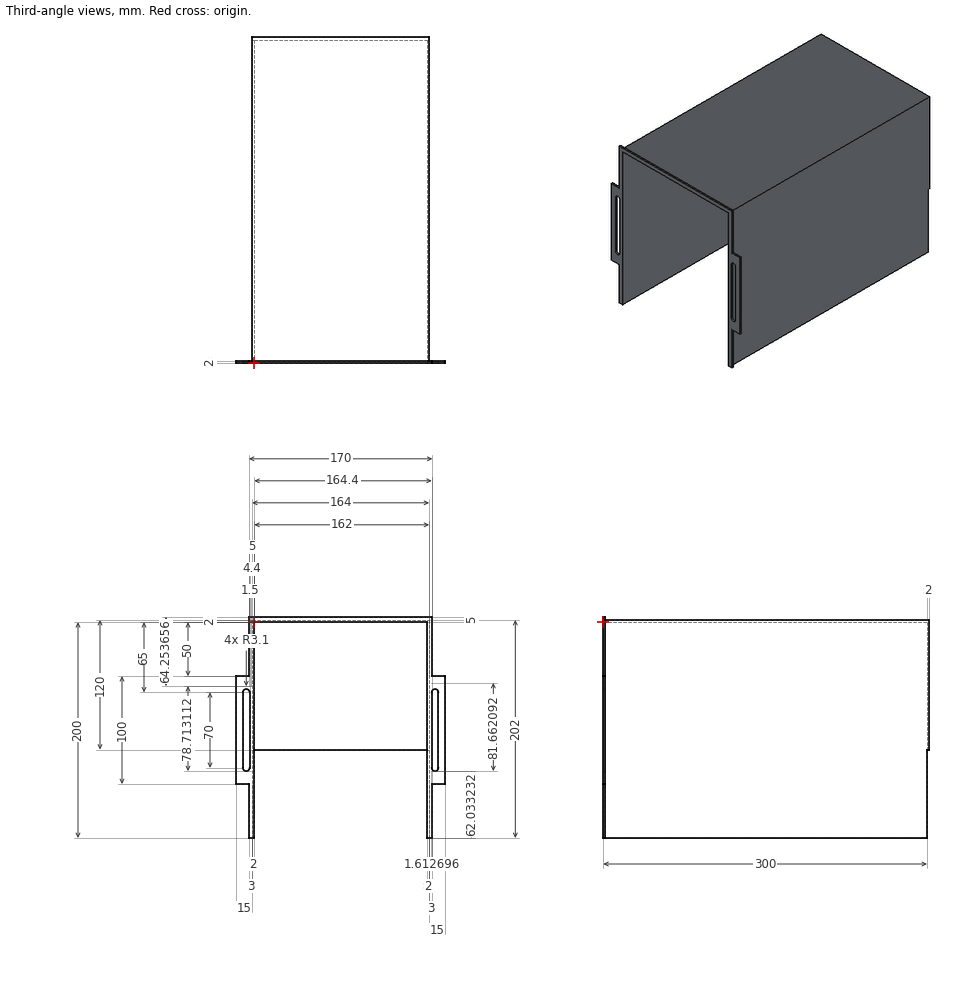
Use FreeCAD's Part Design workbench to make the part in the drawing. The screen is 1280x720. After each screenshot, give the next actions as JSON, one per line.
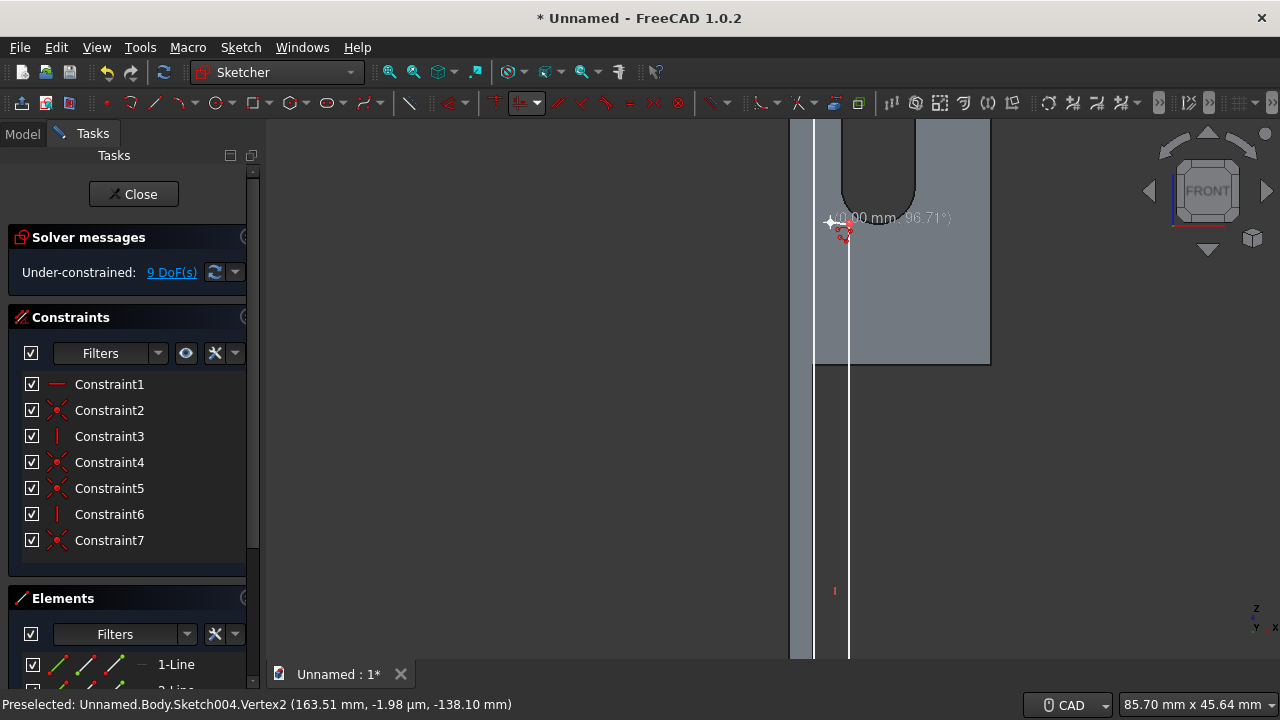
{"action": "scroll", "coordinate": [839, 490], "scroll_direction": "down", "scroll_amount": 10}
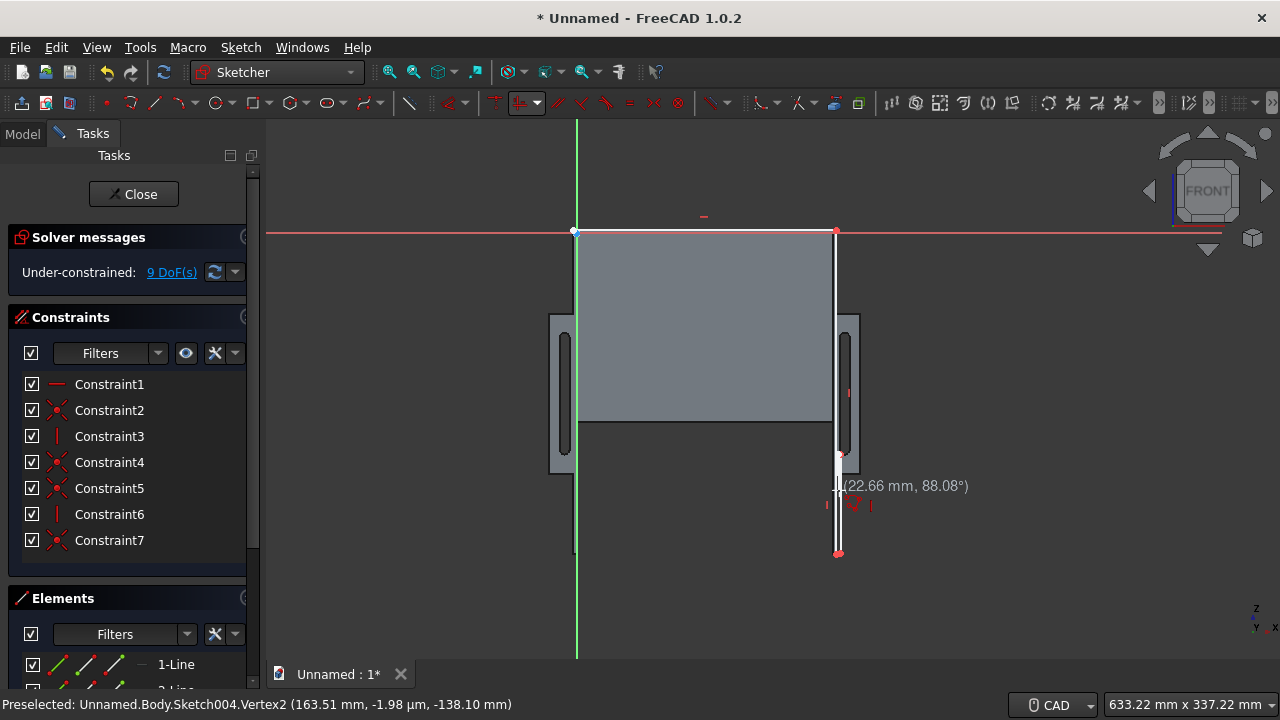
{"action": "scroll", "coordinate": [838, 324], "scroll_direction": "up", "scroll_amount": 10}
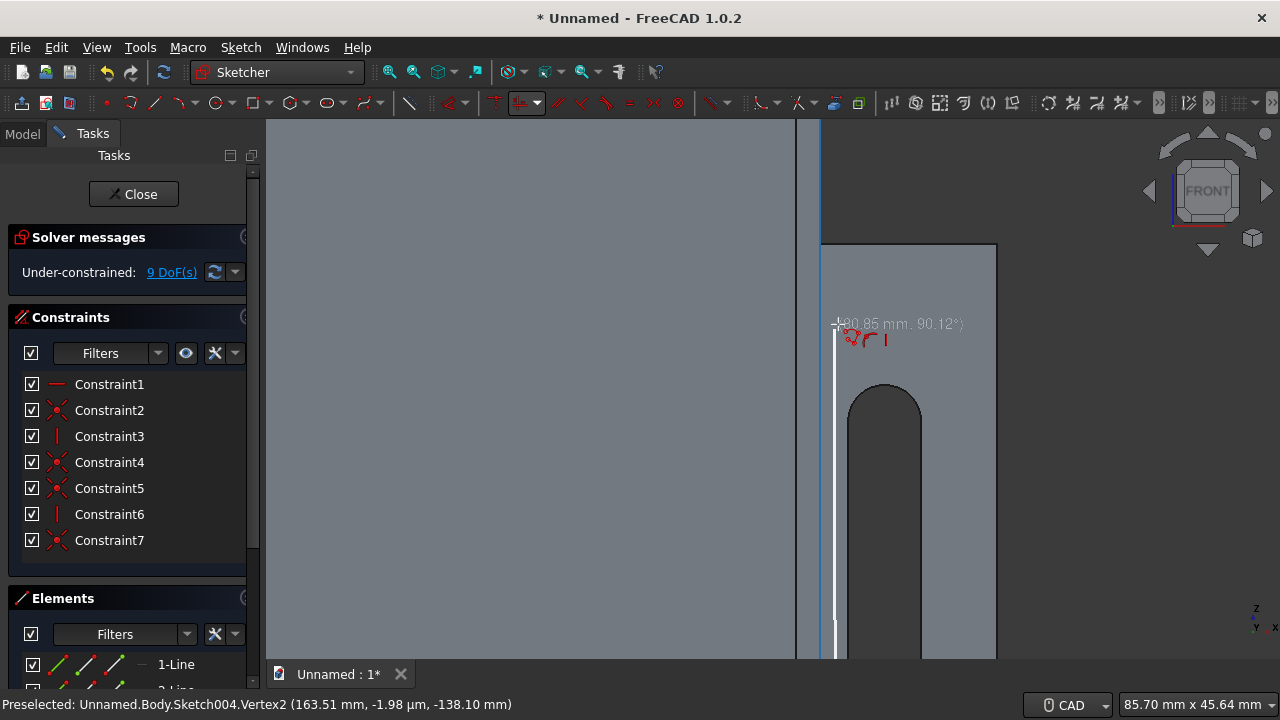
{"action": "left_click", "coordinate": [836, 319]}
{"action": "left_click", "coordinate": [855, 319]}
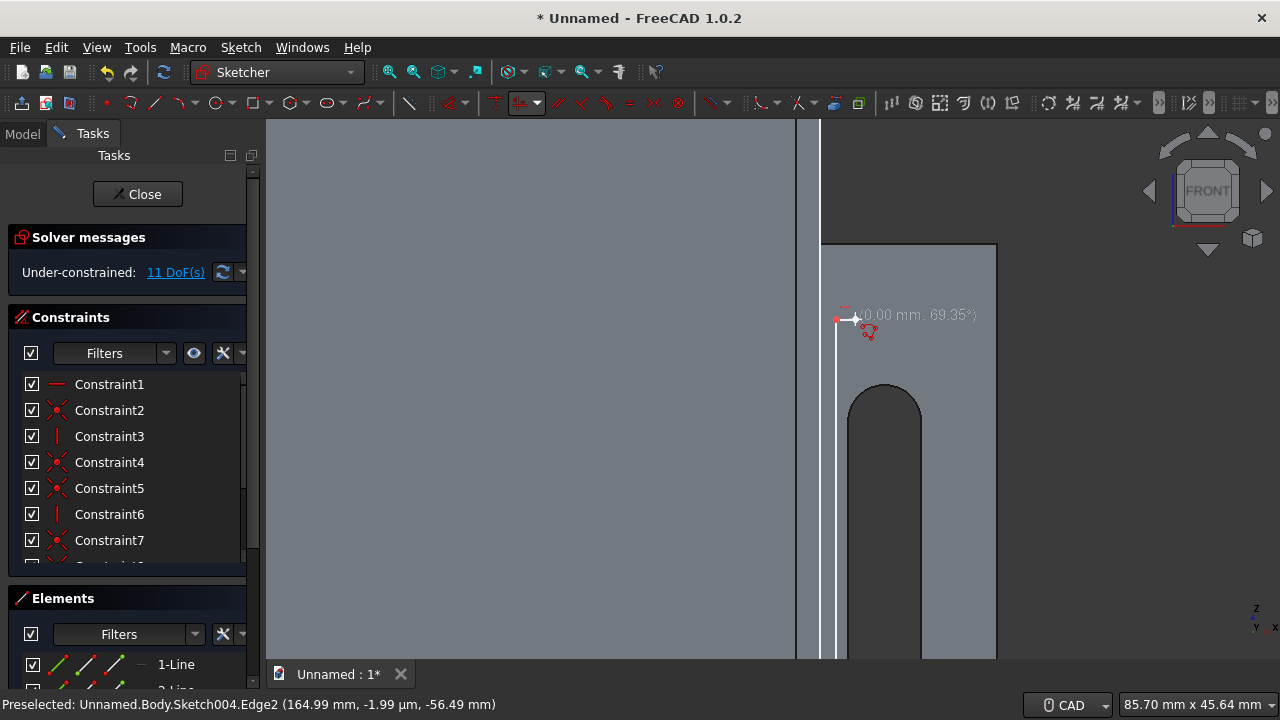
{"action": "scroll", "coordinate": [838, 324], "scroll_direction": "down", "scroll_amount": 10}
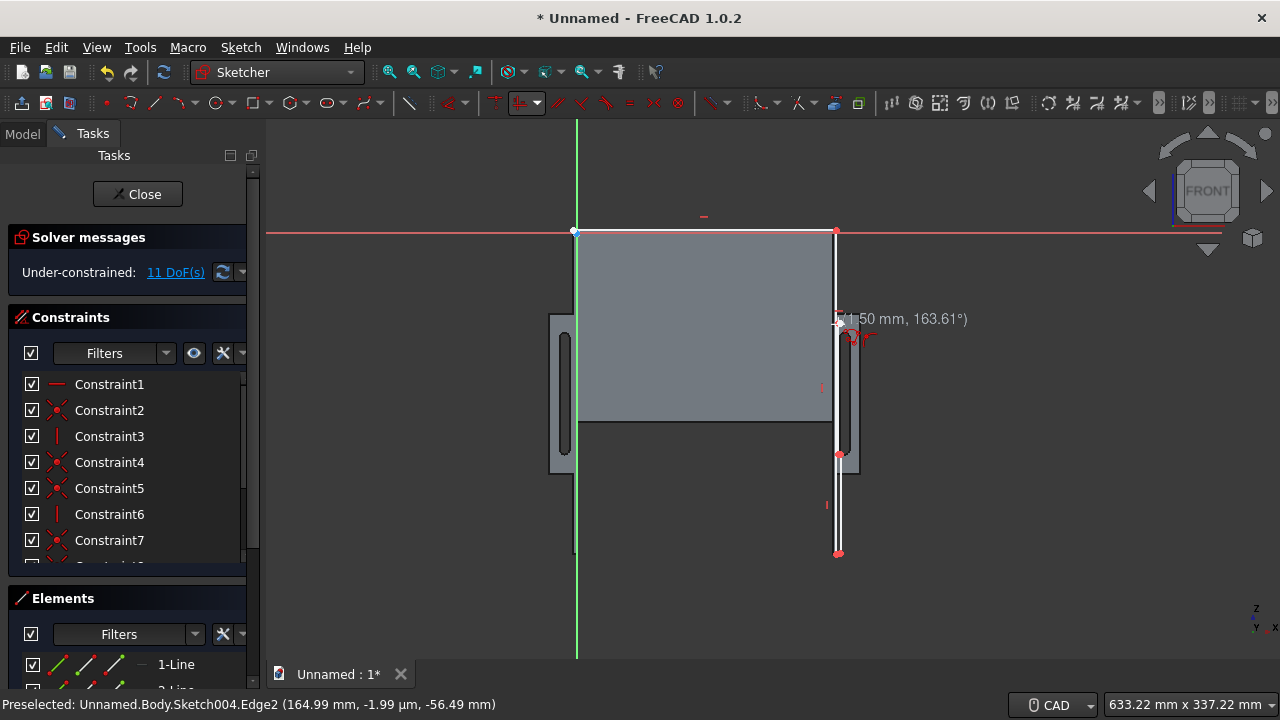
{"action": "scroll", "coordinate": [841, 225], "scroll_direction": "up", "scroll_amount": 5}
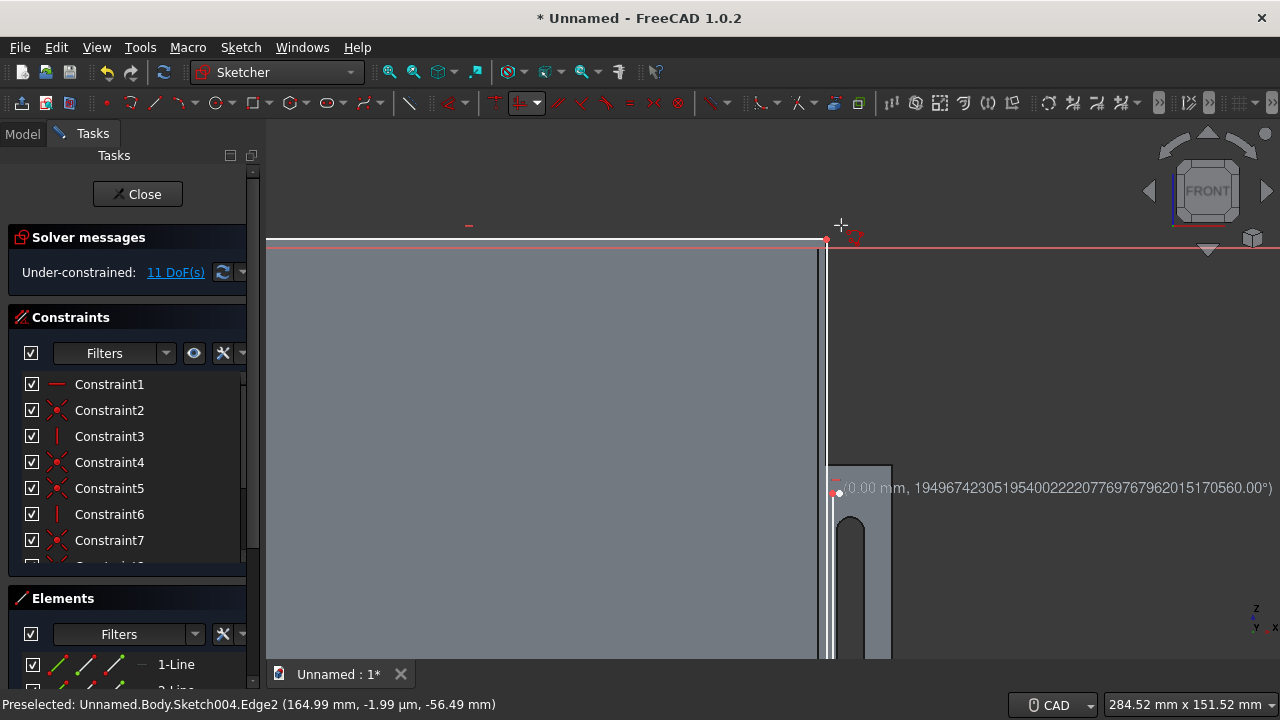
{"action": "left_click", "coordinate": [839, 226]}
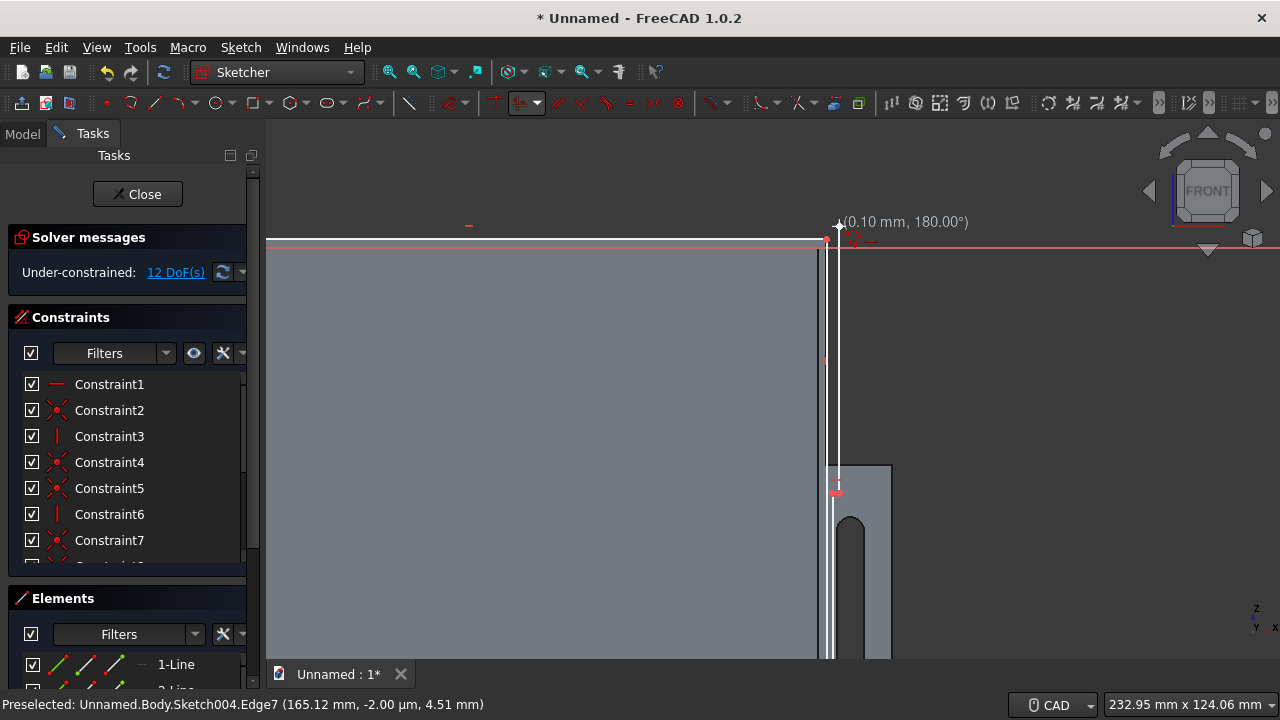
{"action": "scroll", "coordinate": [841, 224], "scroll_direction": "down", "scroll_amount": 5}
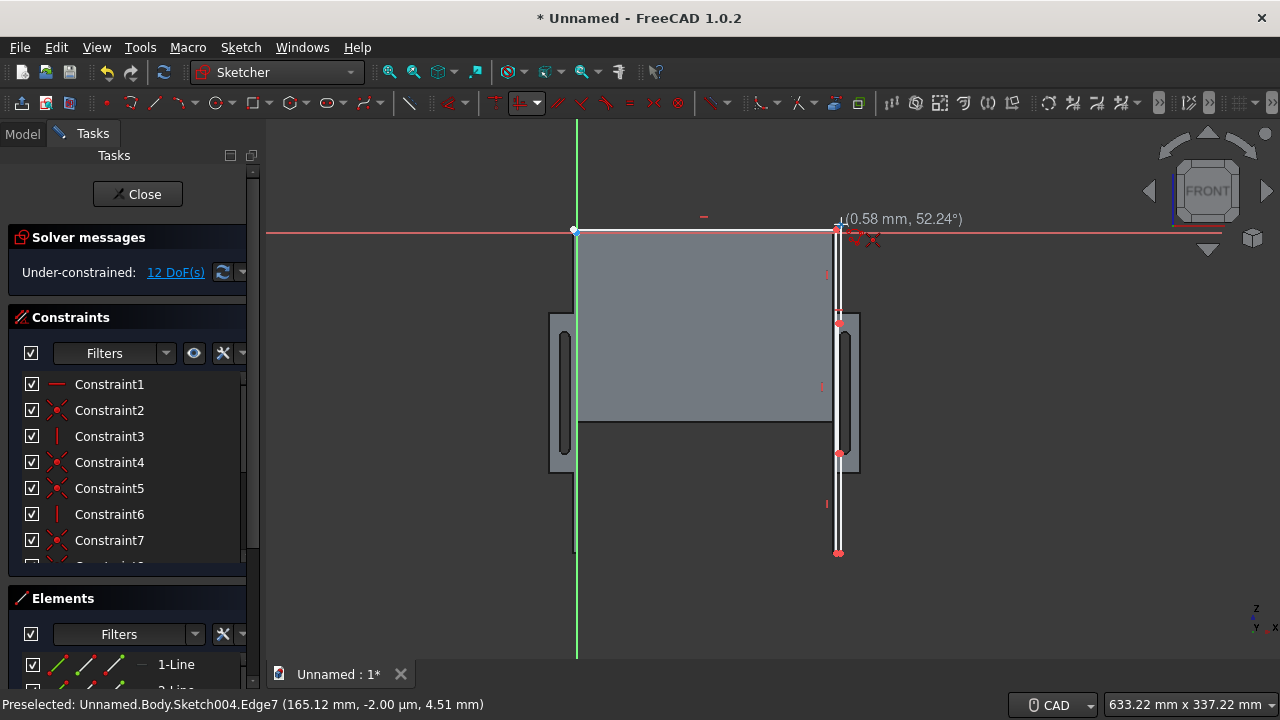
{"action": "scroll", "coordinate": [569, 225], "scroll_direction": "up", "scroll_amount": 5}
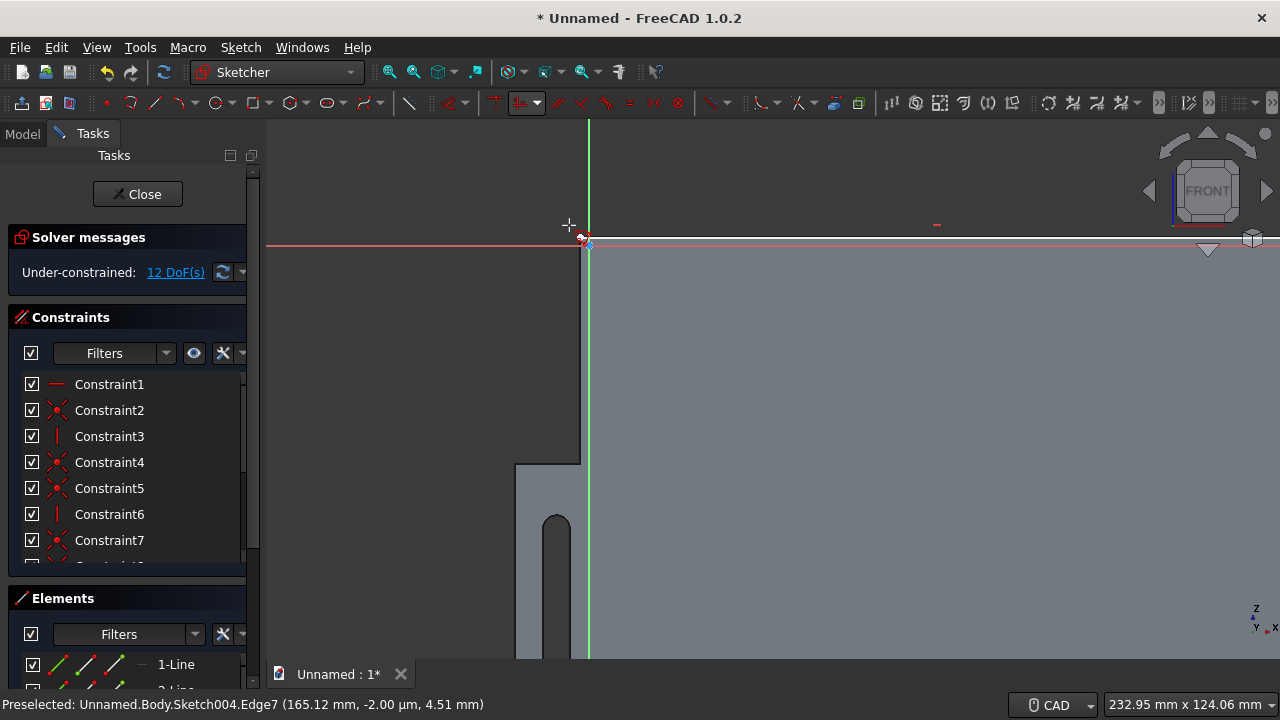
{"action": "left_click", "coordinate": [567, 224]}
{"action": "left_click", "coordinate": [567, 504]}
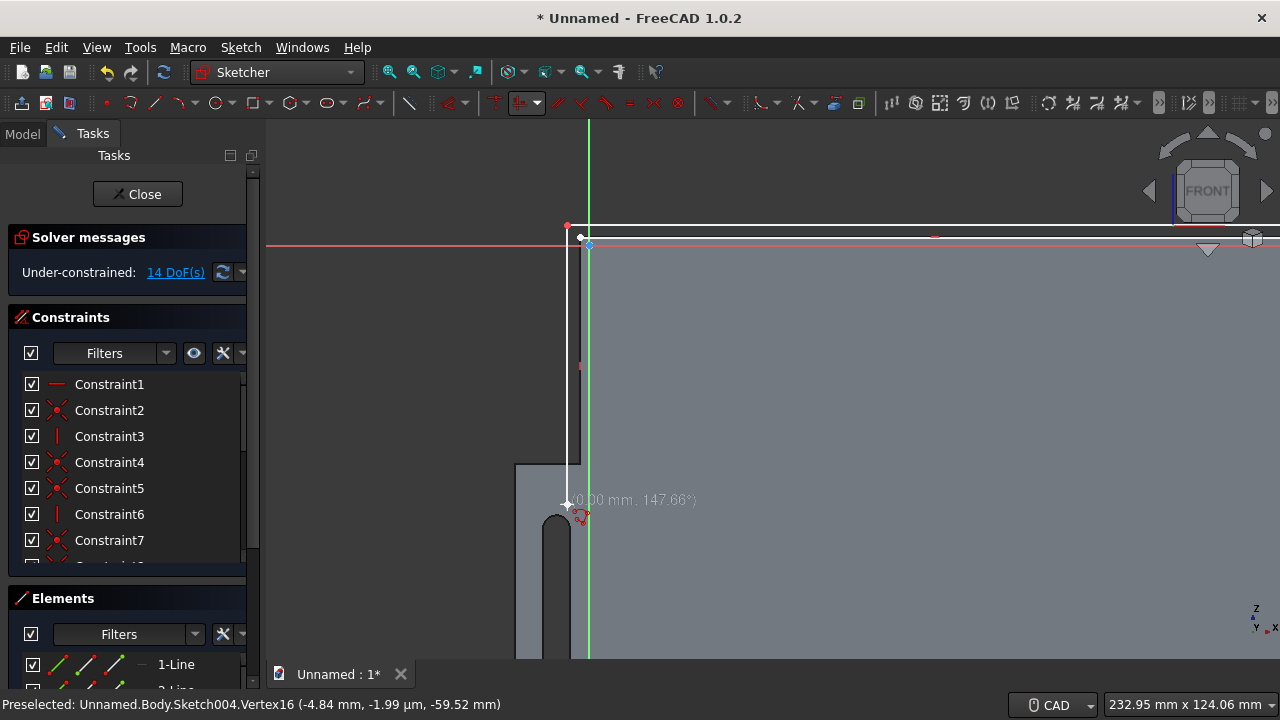
{"action": "scroll", "coordinate": [574, 504], "scroll_direction": "up", "scroll_amount": 5}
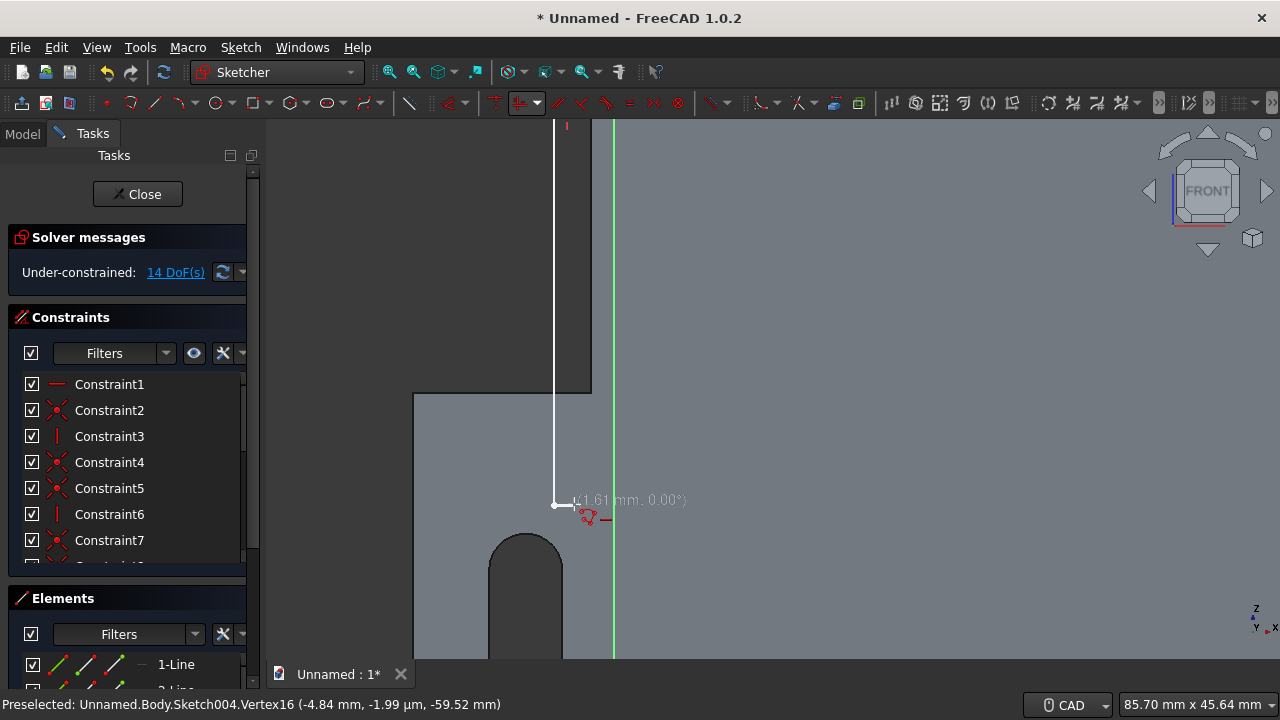
{"action": "left_click", "coordinate": [573, 503]}